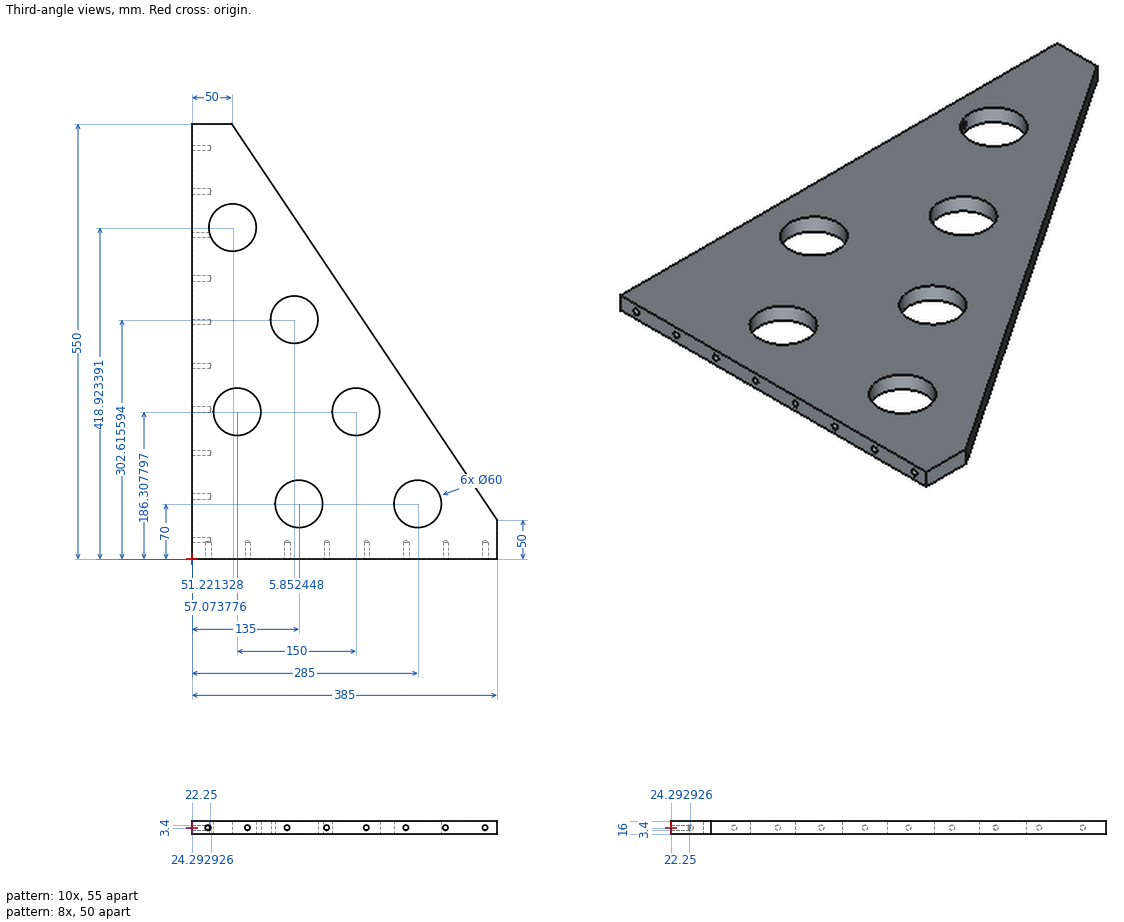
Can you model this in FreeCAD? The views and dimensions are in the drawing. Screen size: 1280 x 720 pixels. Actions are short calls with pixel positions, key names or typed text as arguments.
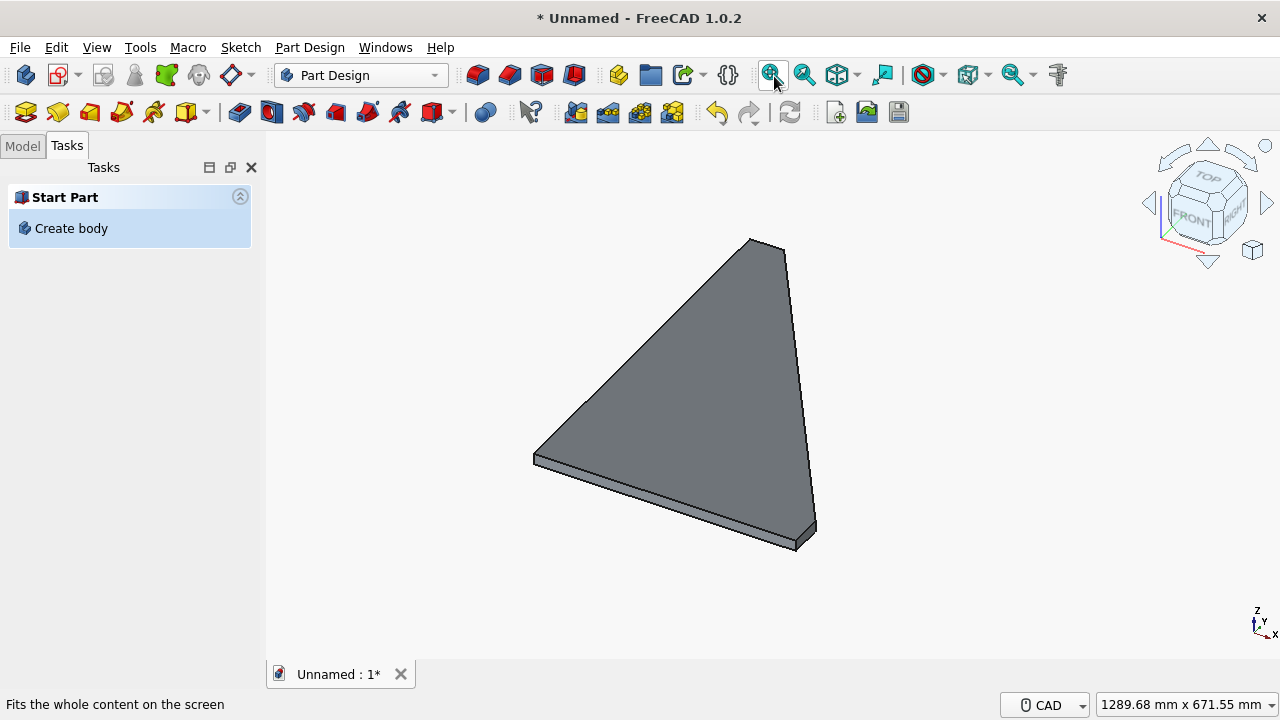
click(23, 145)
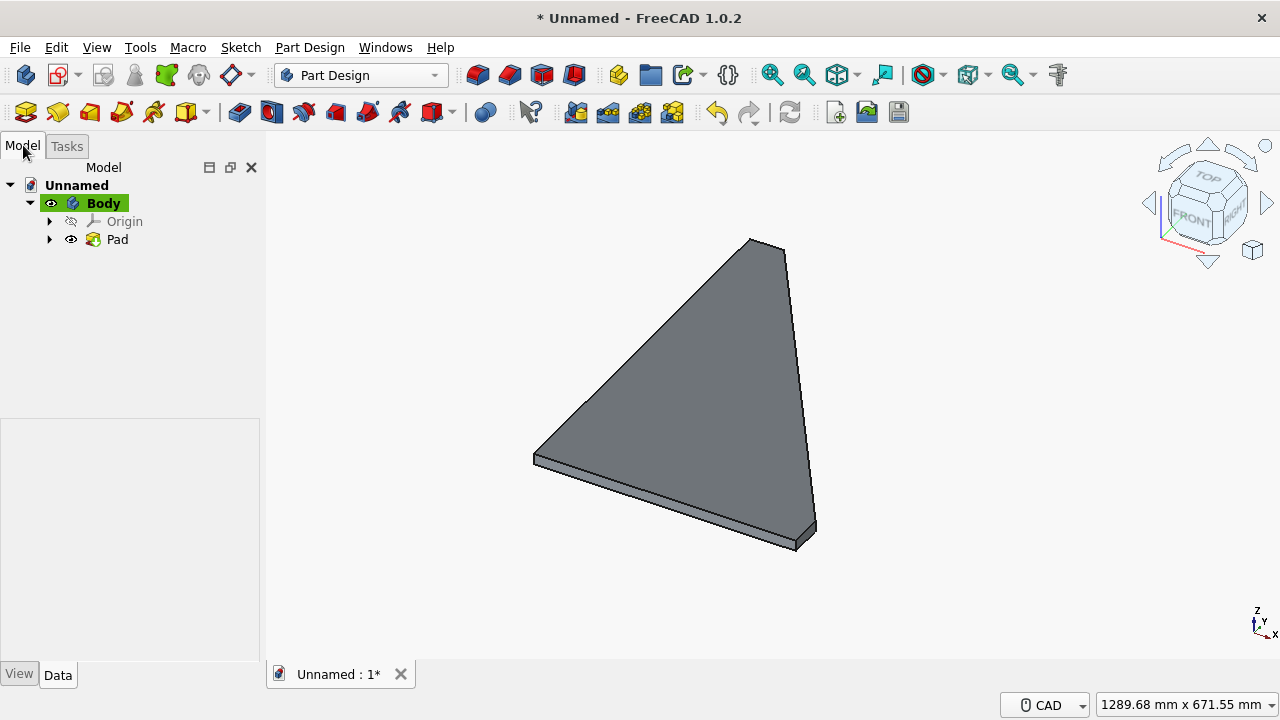
click(50, 221)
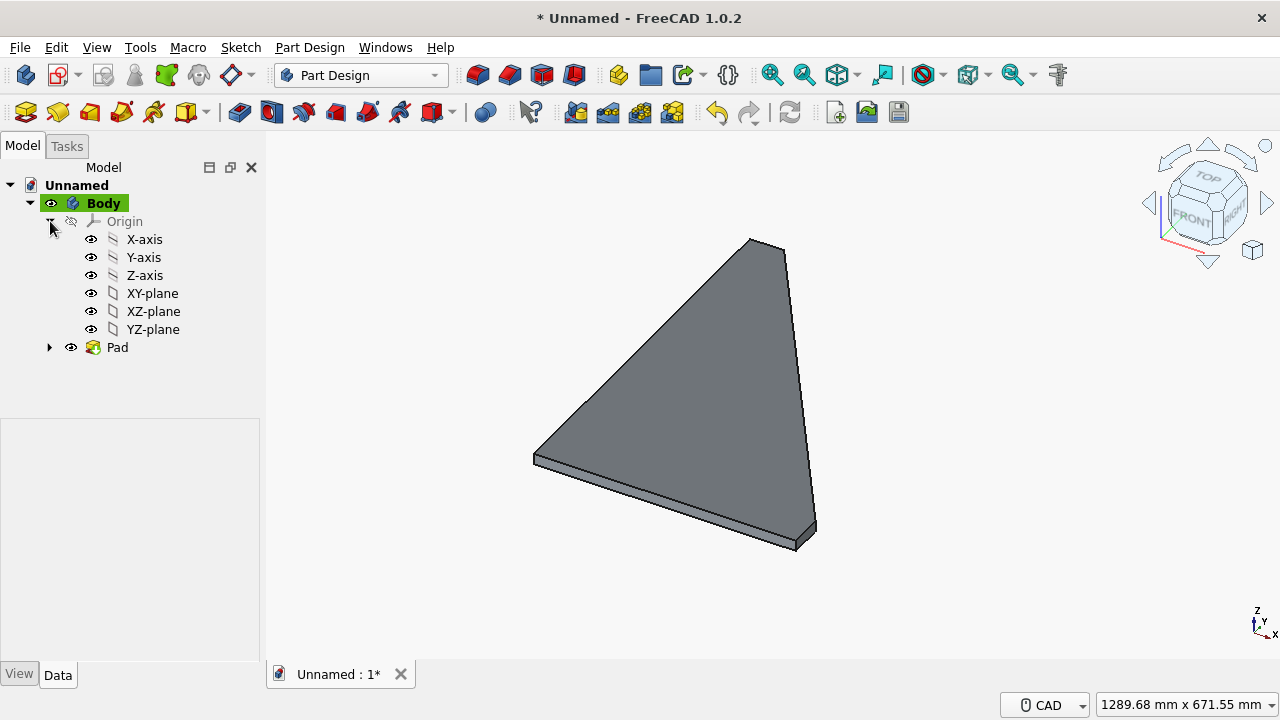
click(136, 311)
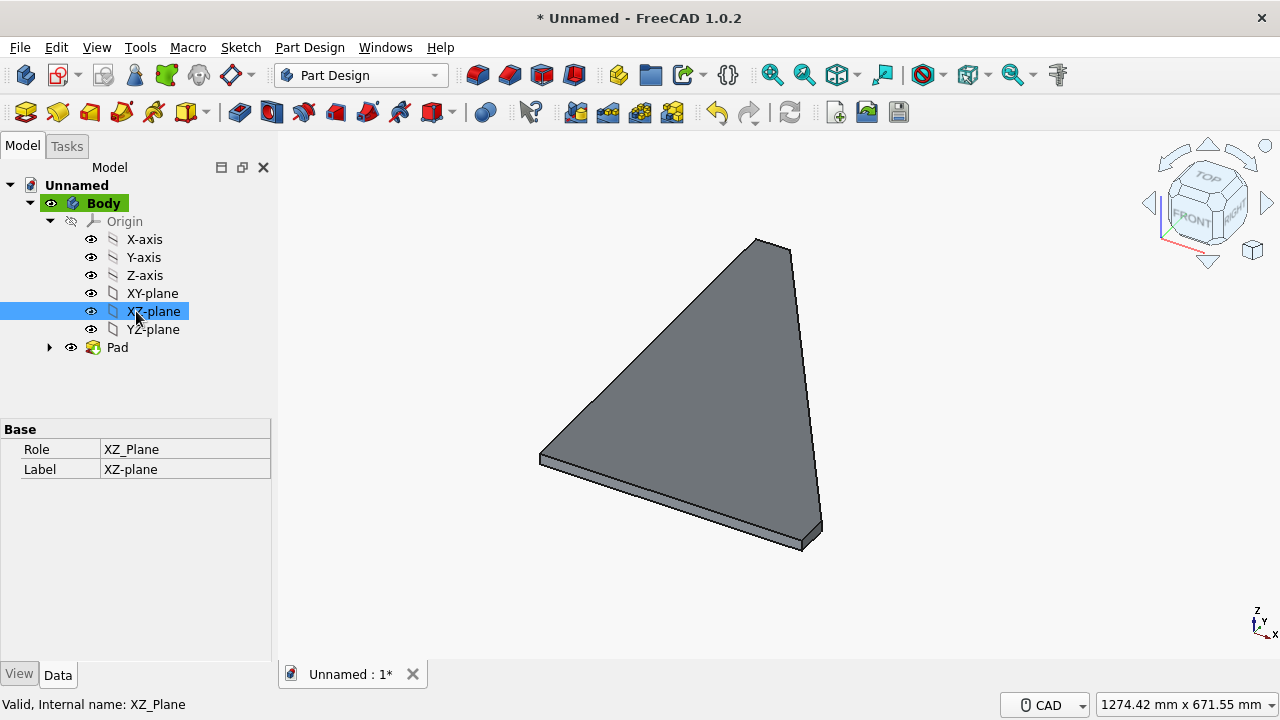
click(232, 76)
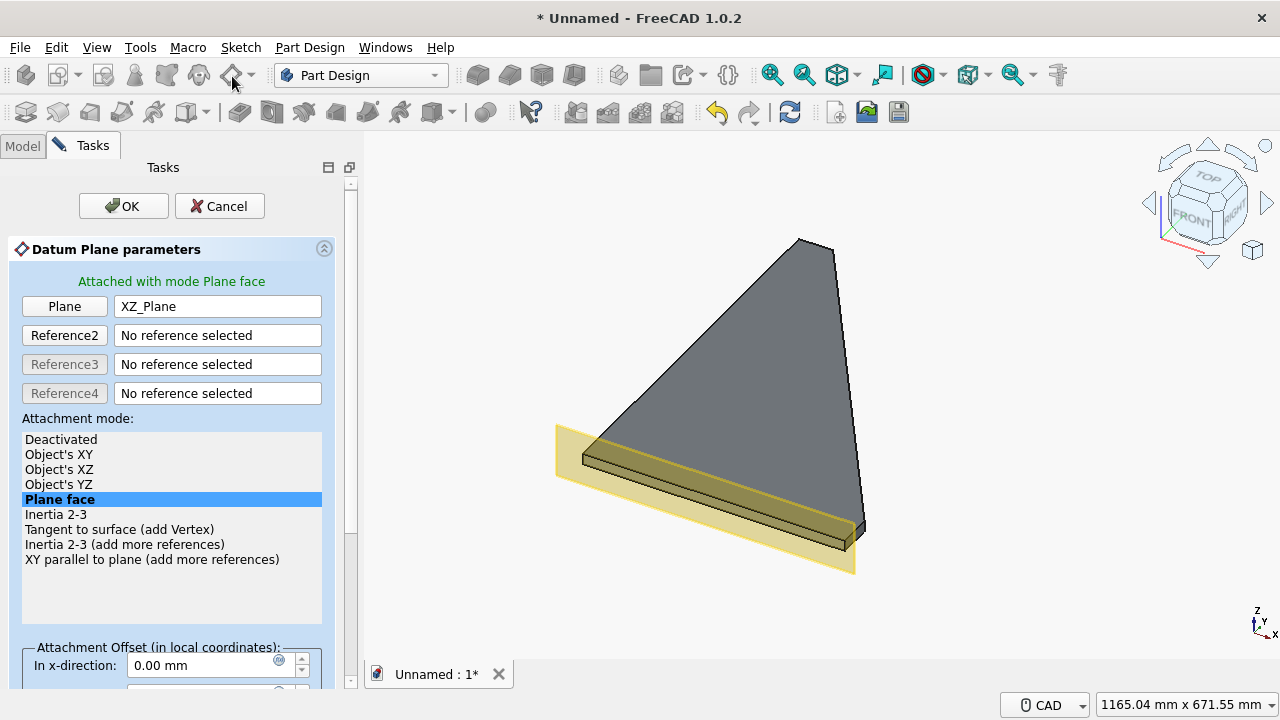
scroll(351, 432, down, 2)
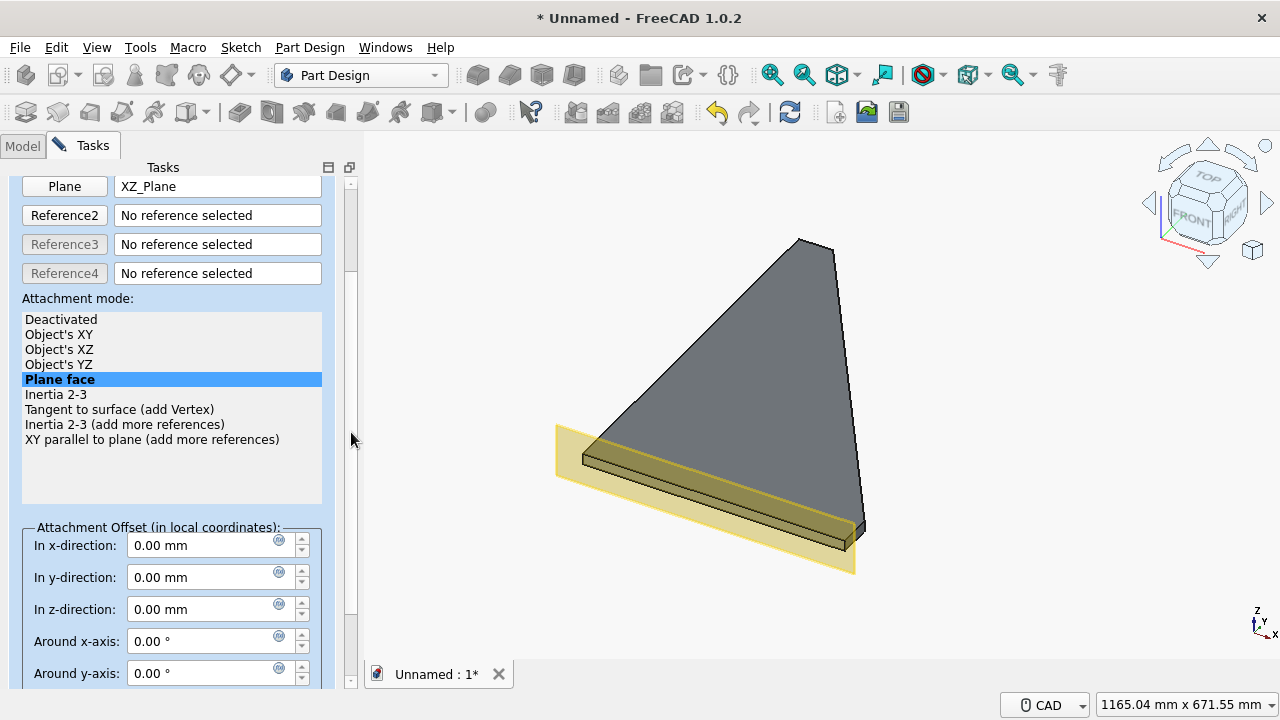
triple_click(210, 609)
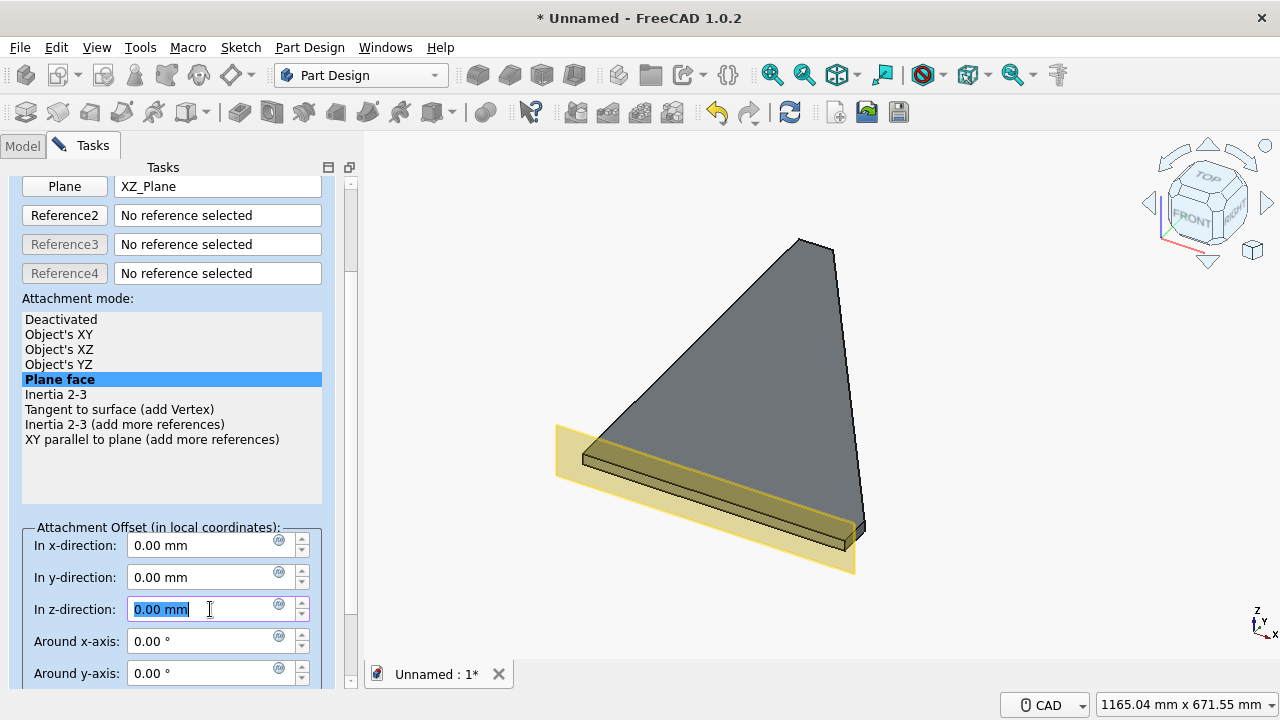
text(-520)
key(Tab)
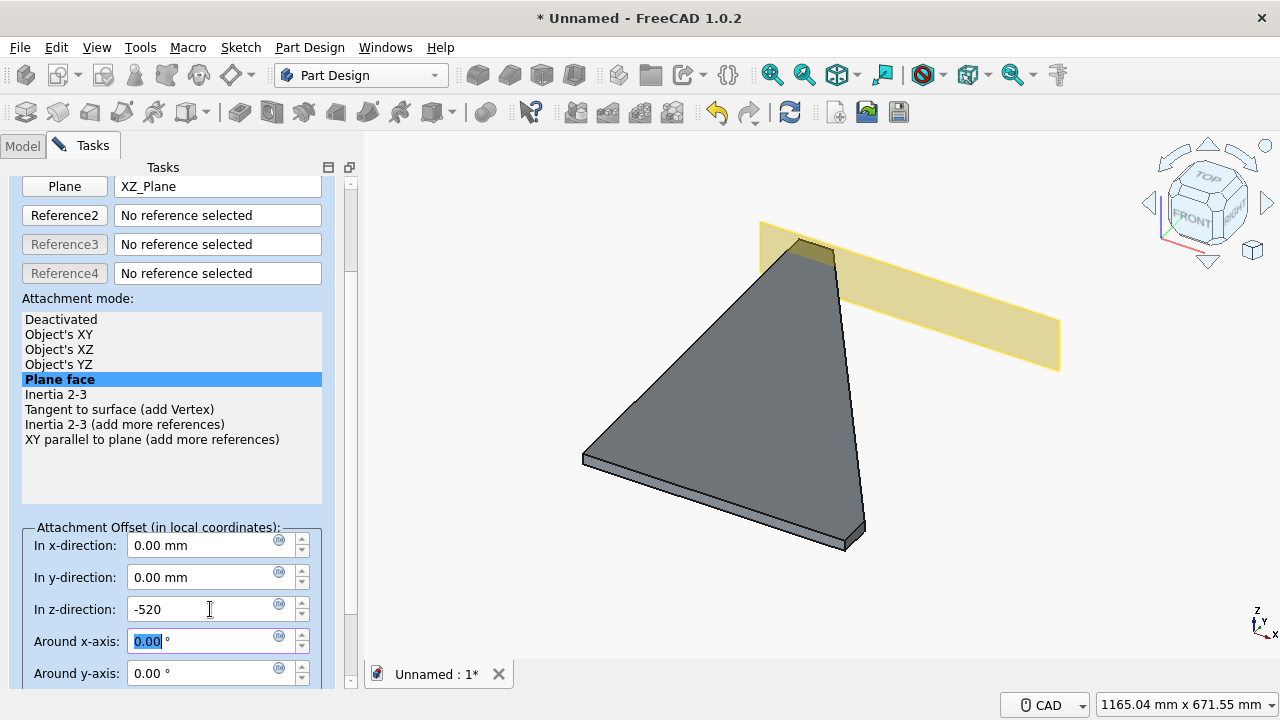
scroll(351, 432, up, 3)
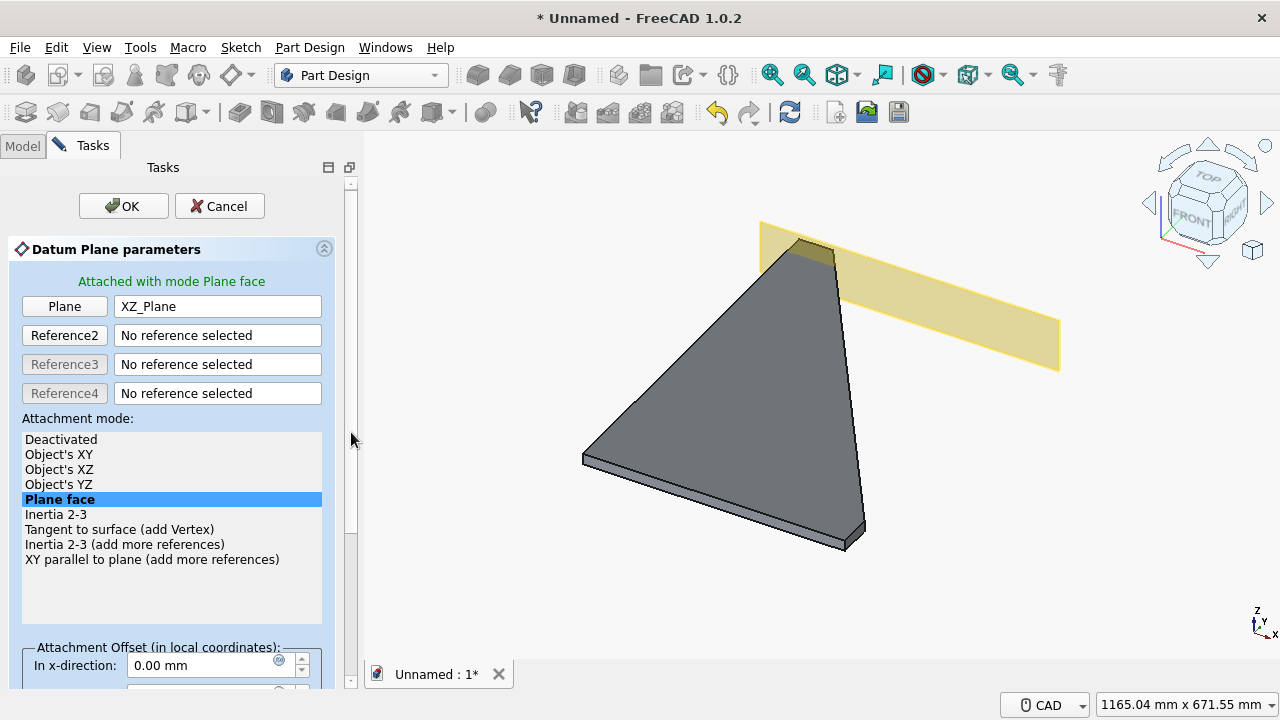
click(124, 206)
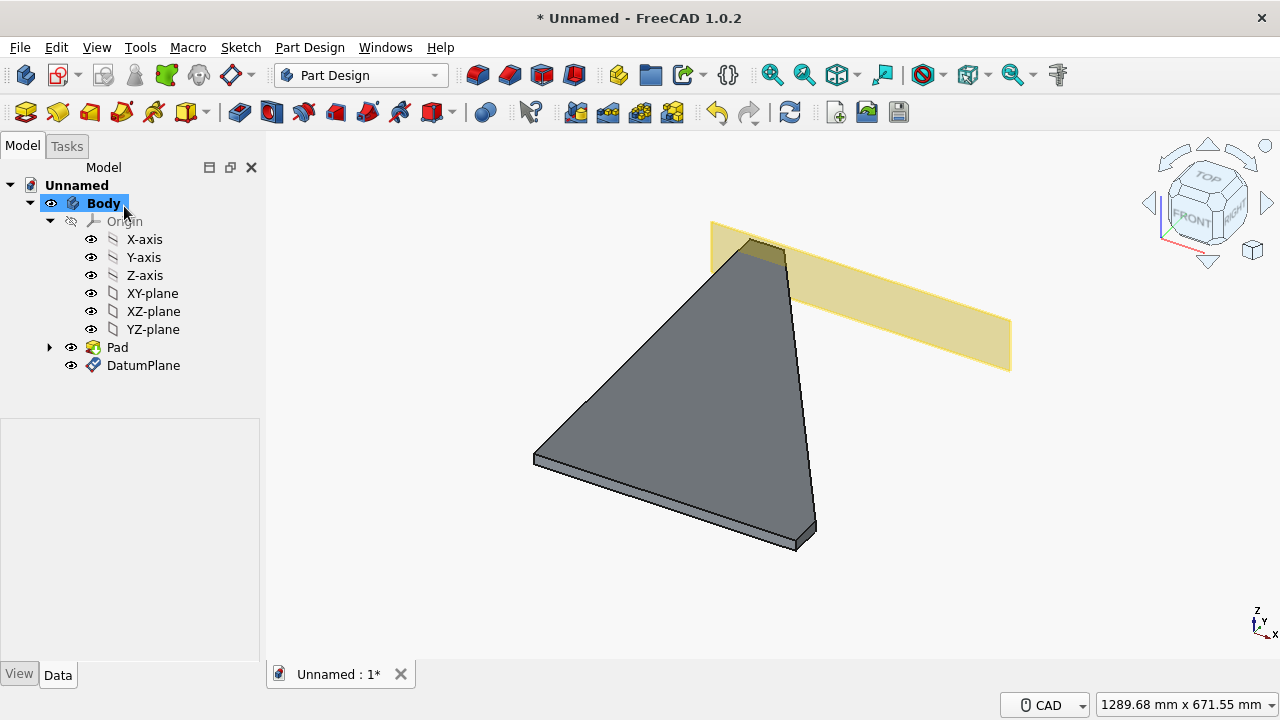
click(116, 365)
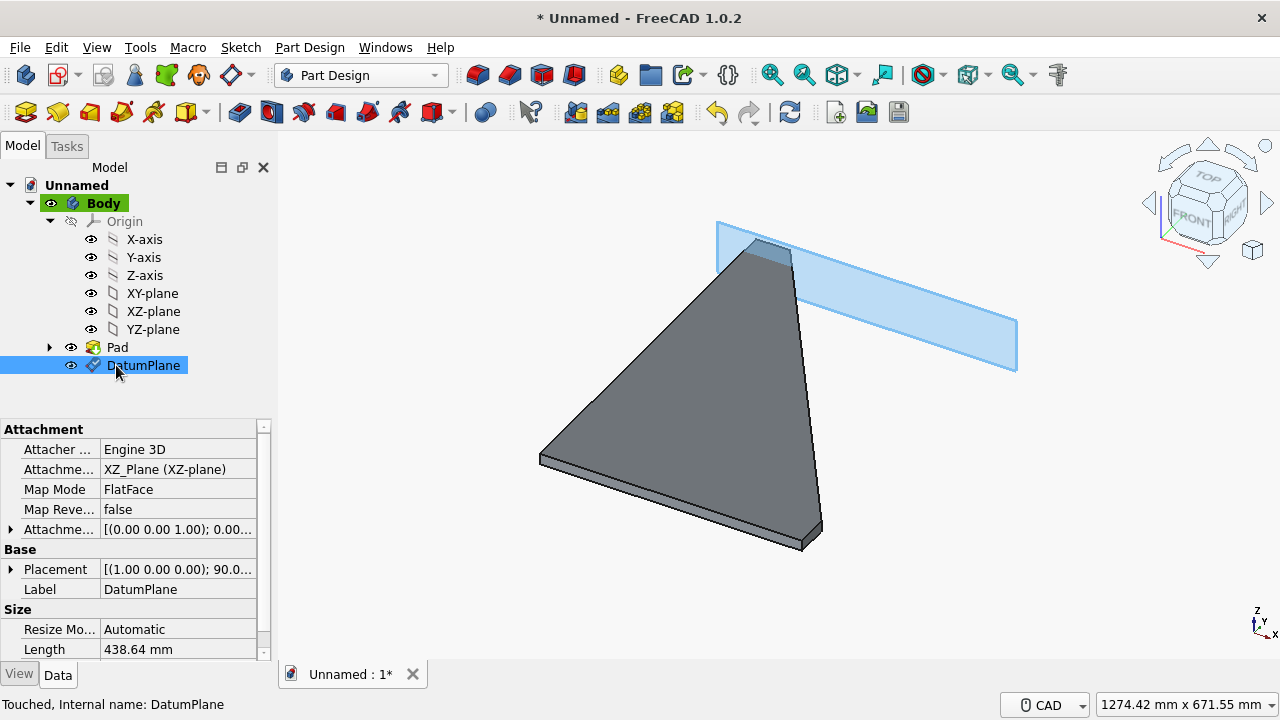
click(58, 76)